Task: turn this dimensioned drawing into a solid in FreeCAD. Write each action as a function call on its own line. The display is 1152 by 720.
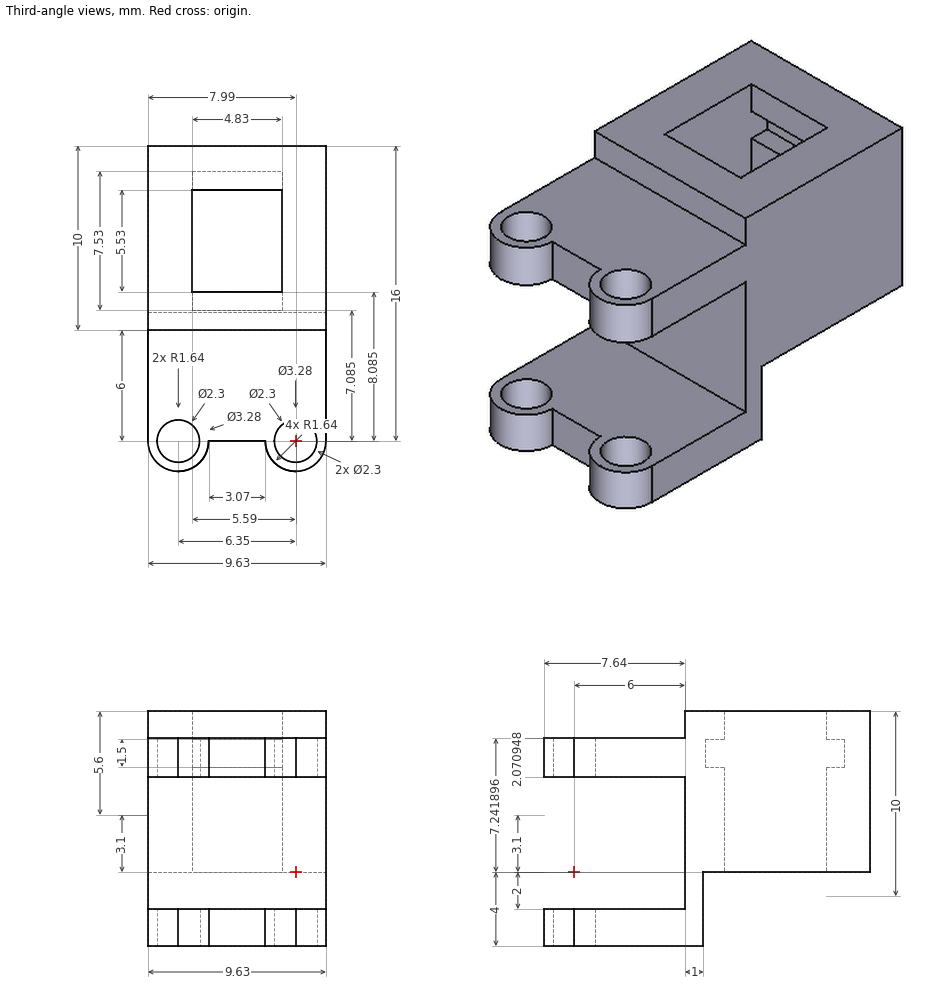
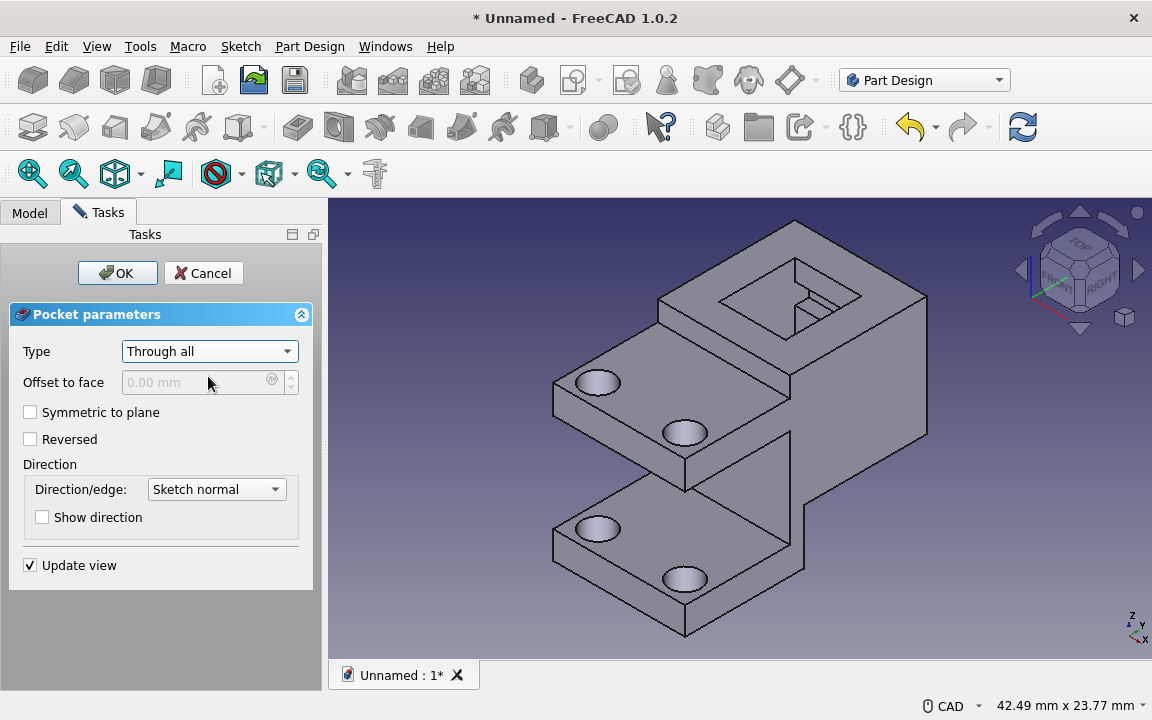
click(118, 273)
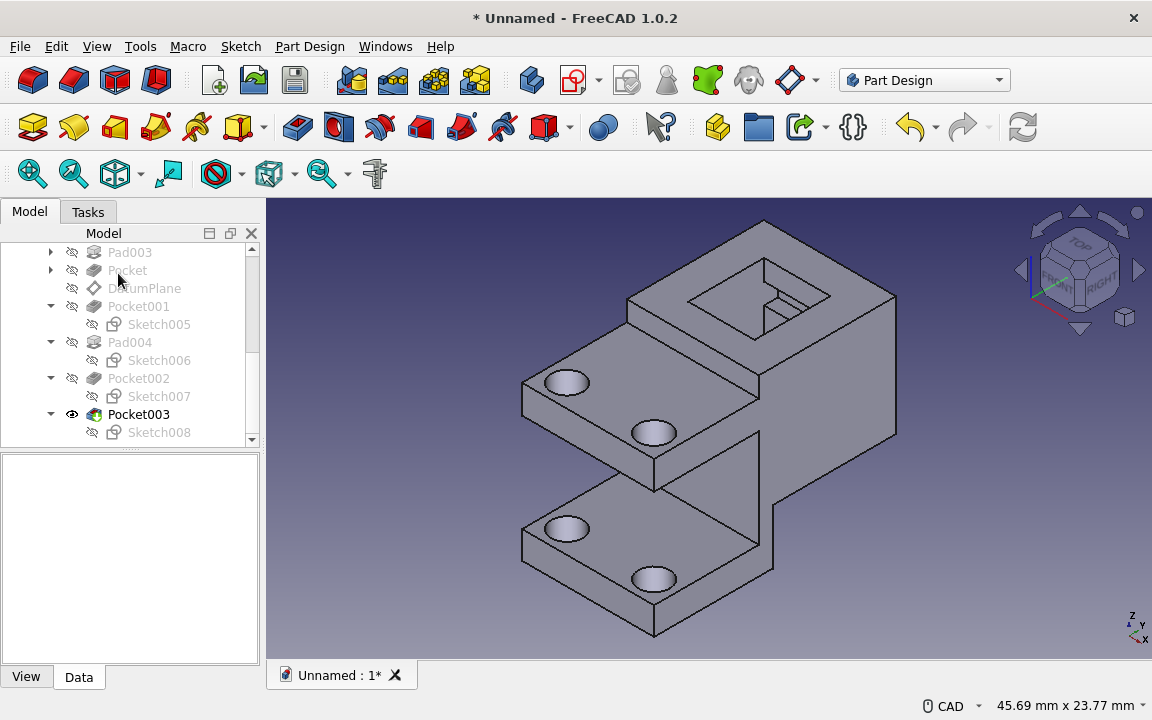
key(5)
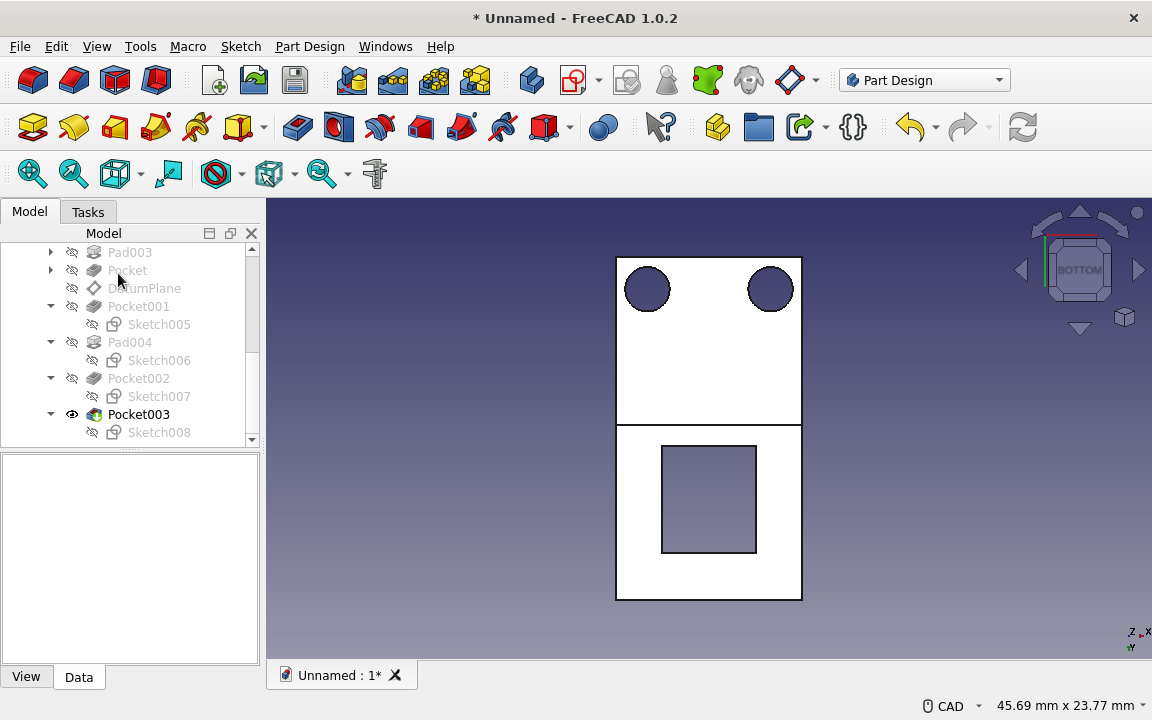
click(736, 364)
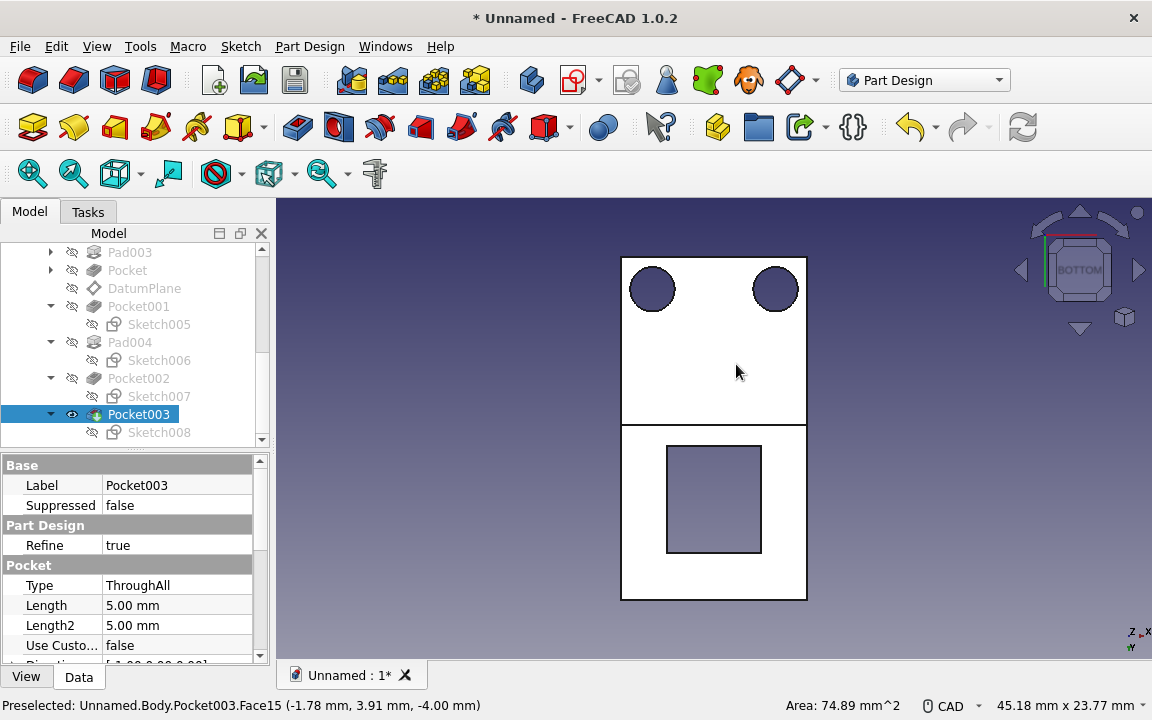
click(572, 80)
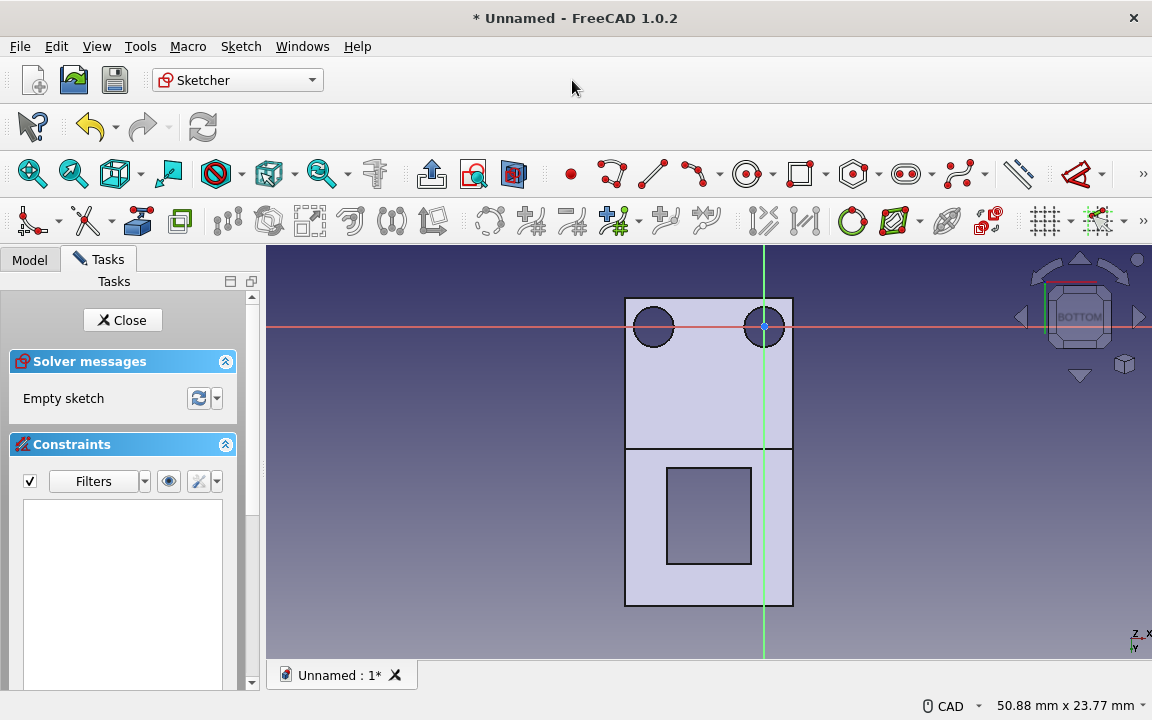
scroll(749, 273, up, 5)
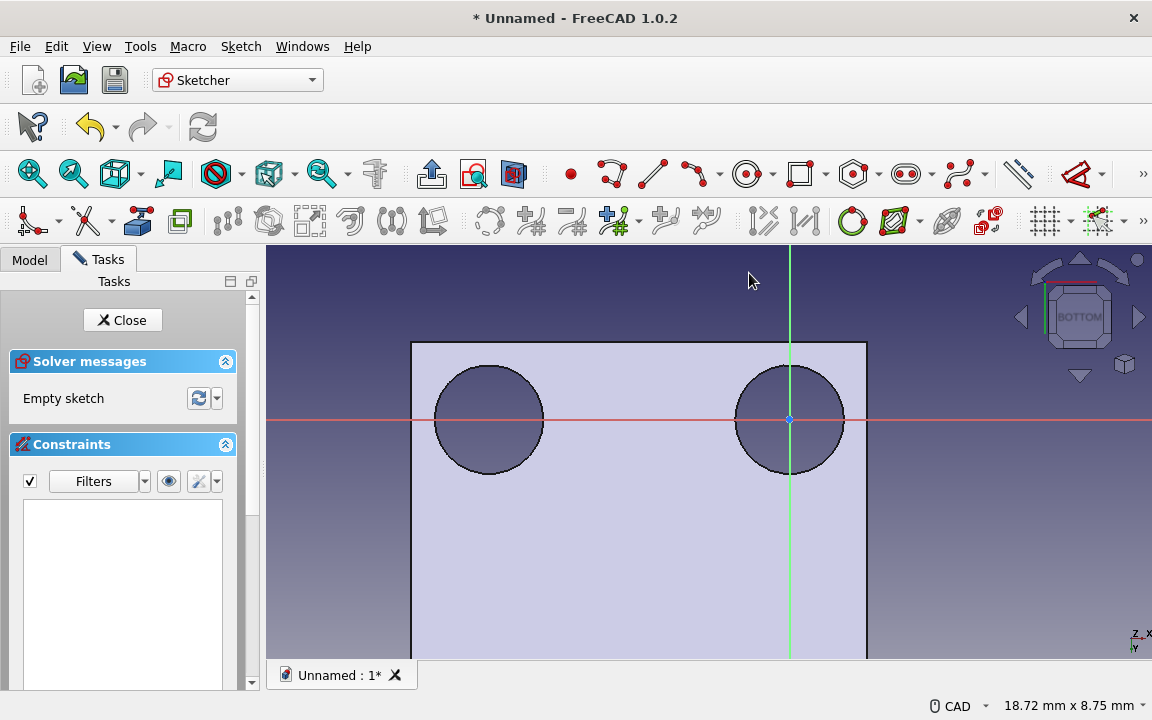
click(653, 174)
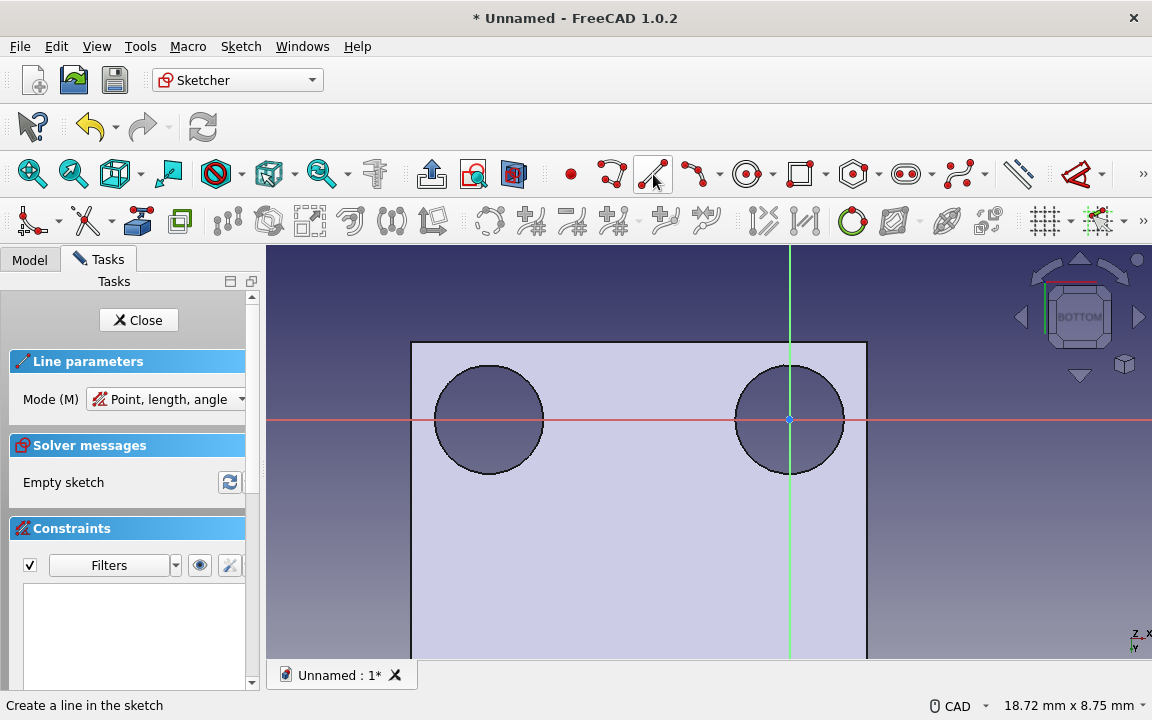
click(567, 420)
click(712, 411)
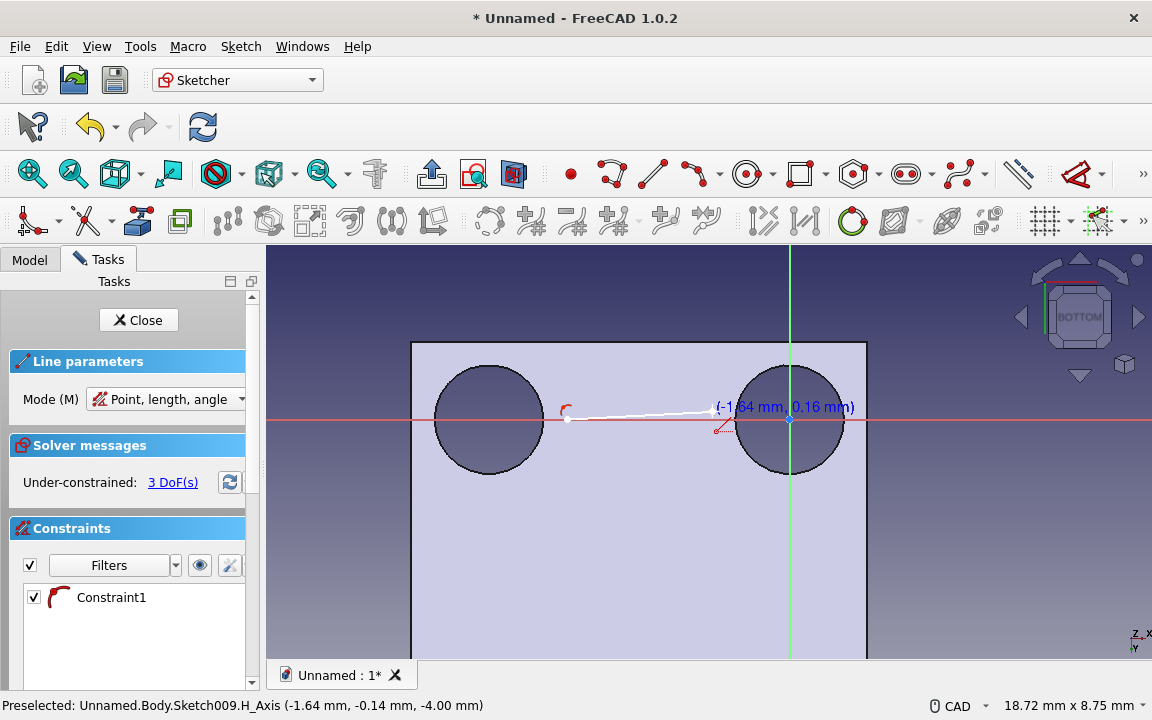
click(790, 342)
click(489, 342)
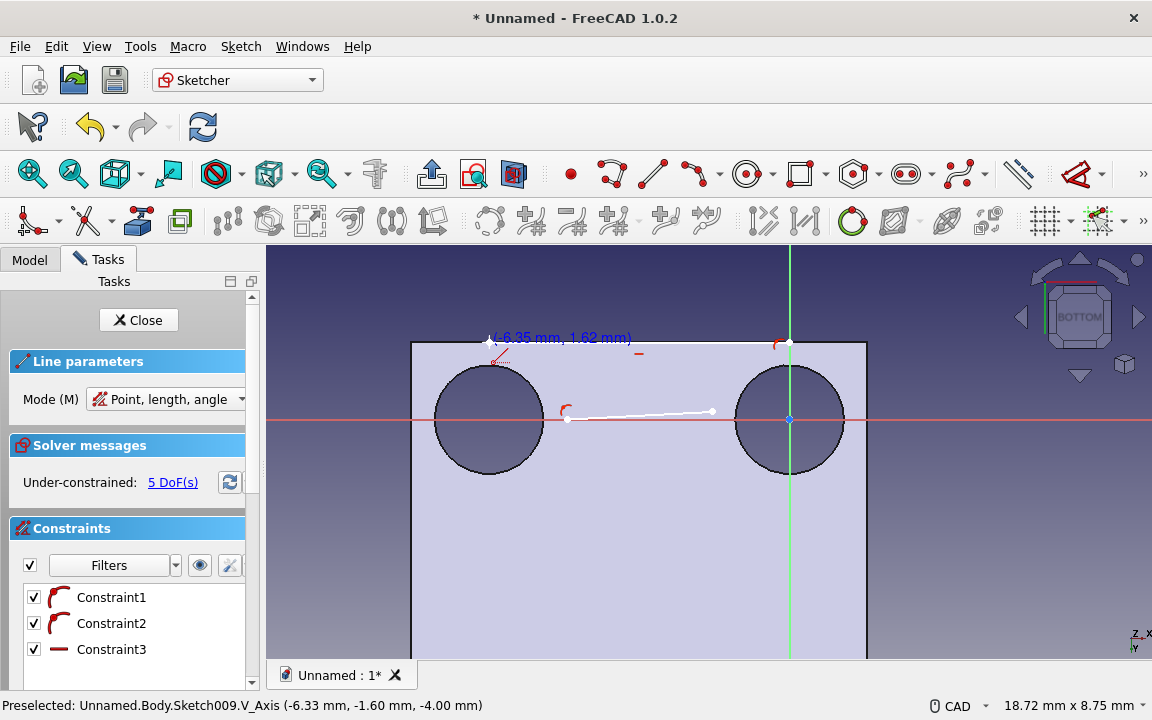
click(694, 174)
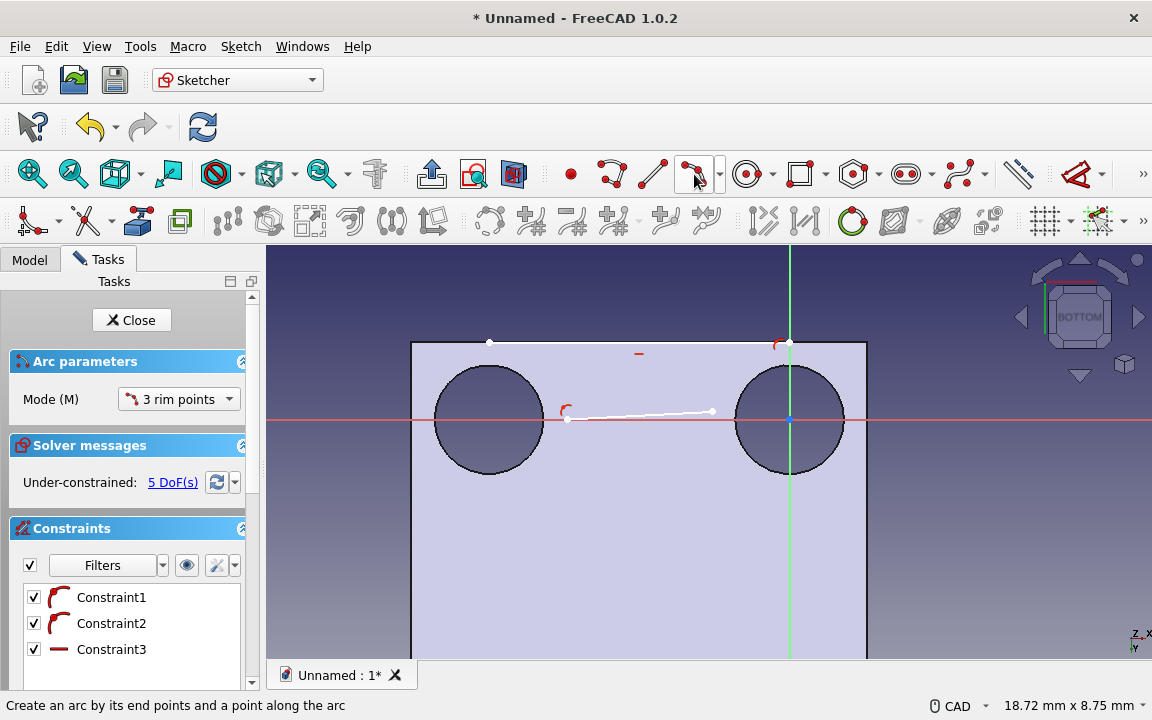
click(712, 412)
click(790, 343)
click(735, 365)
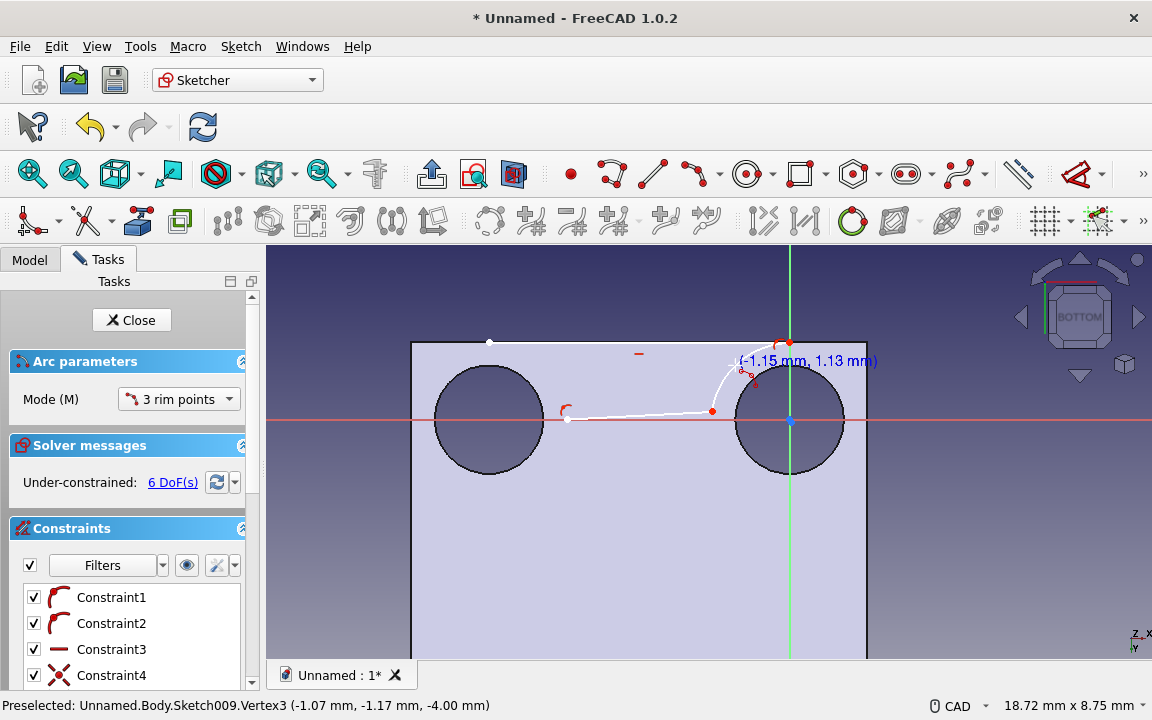
click(489, 343)
click(567, 420)
click(544, 365)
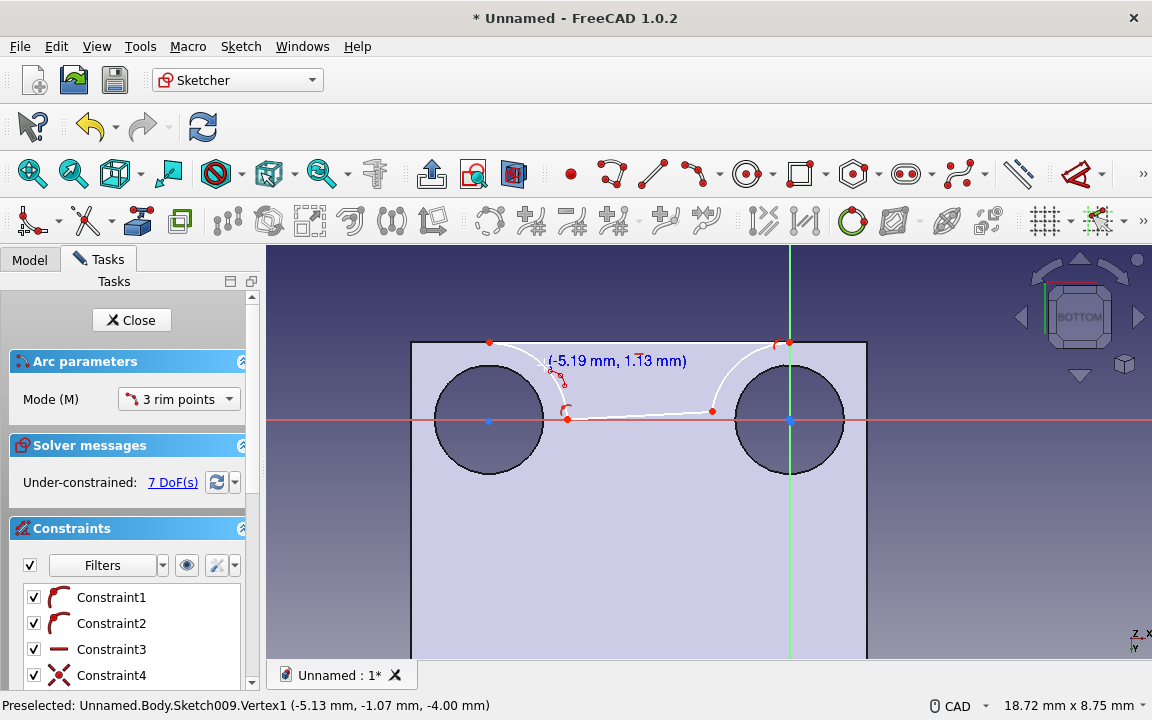
click(612, 174)